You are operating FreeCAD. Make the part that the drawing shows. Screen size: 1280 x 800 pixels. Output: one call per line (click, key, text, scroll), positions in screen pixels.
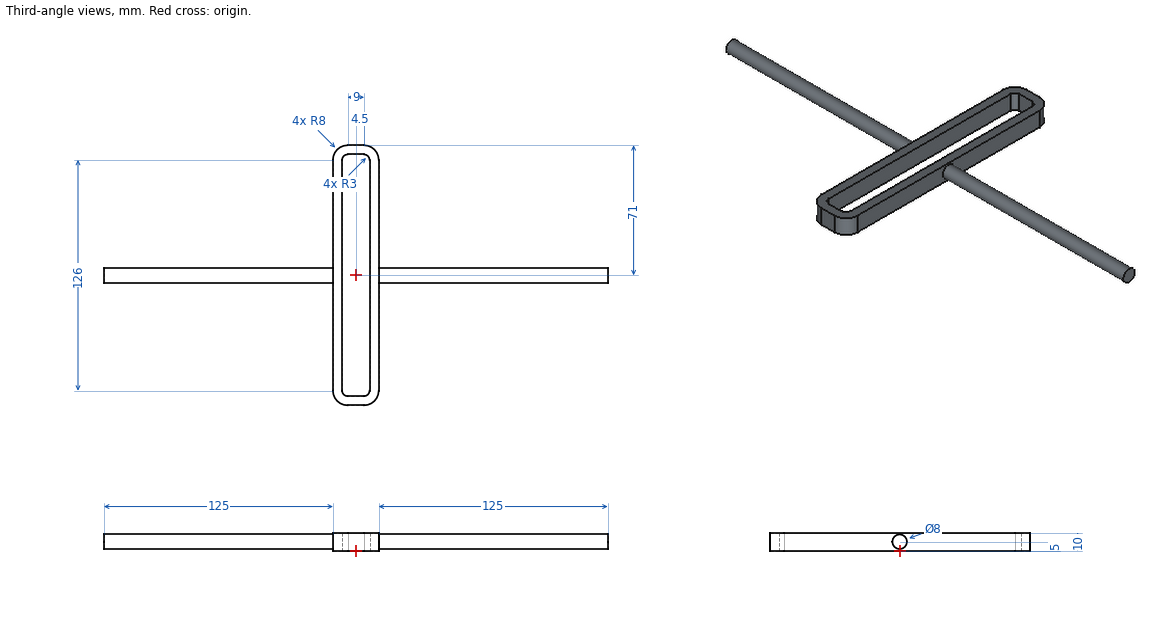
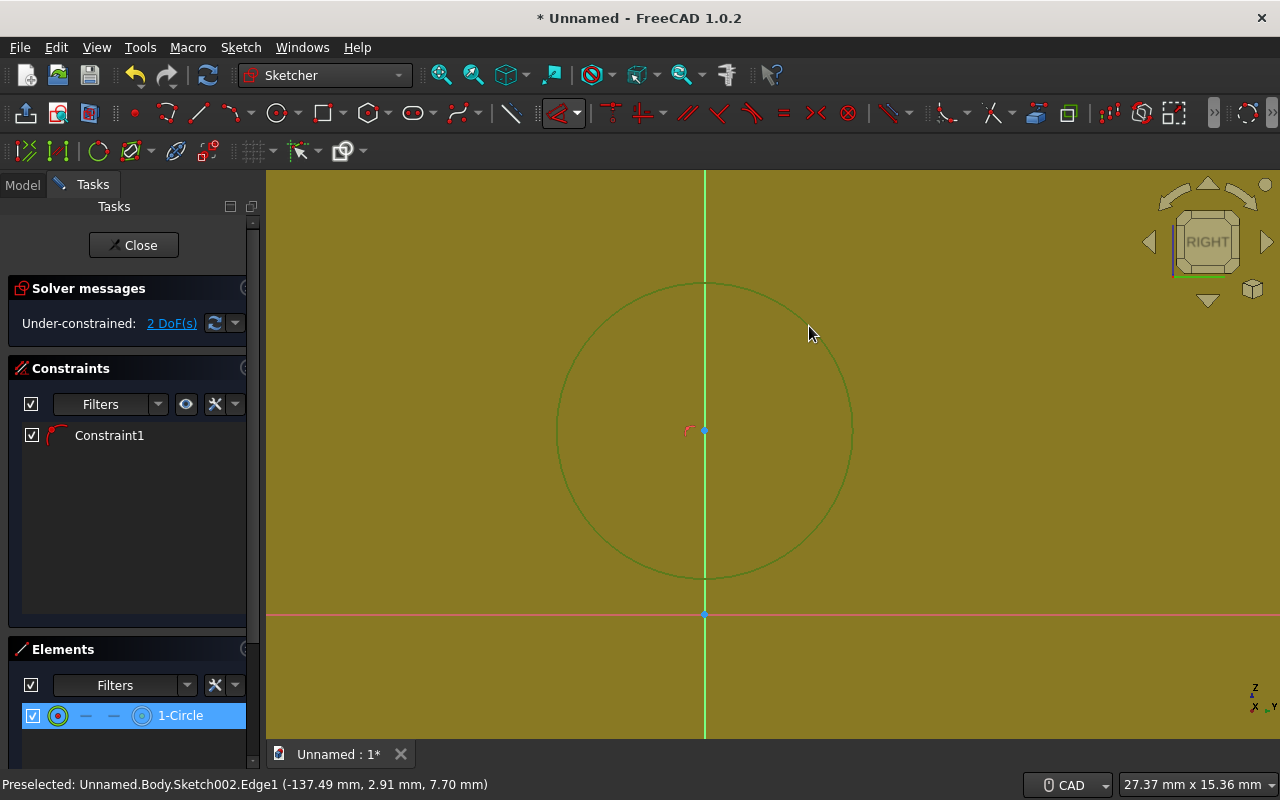
click(580, 114)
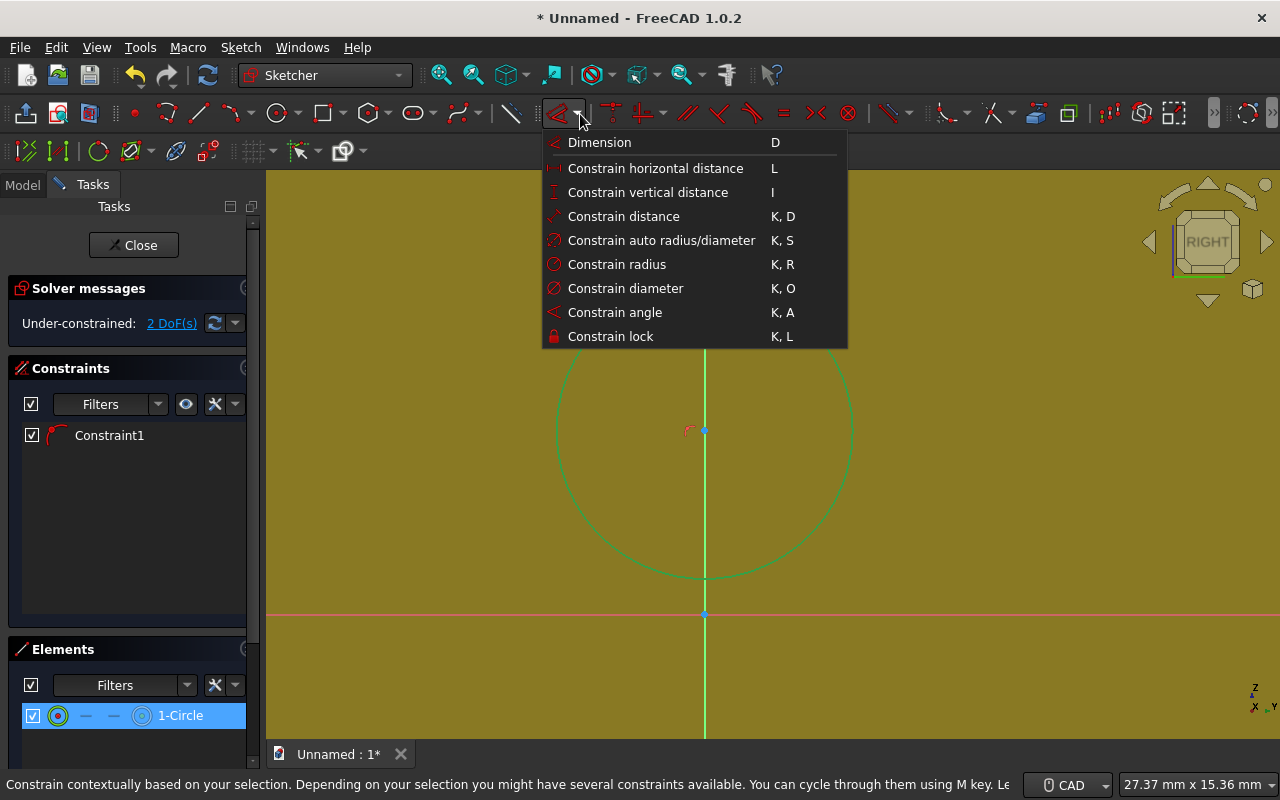
click(695, 288)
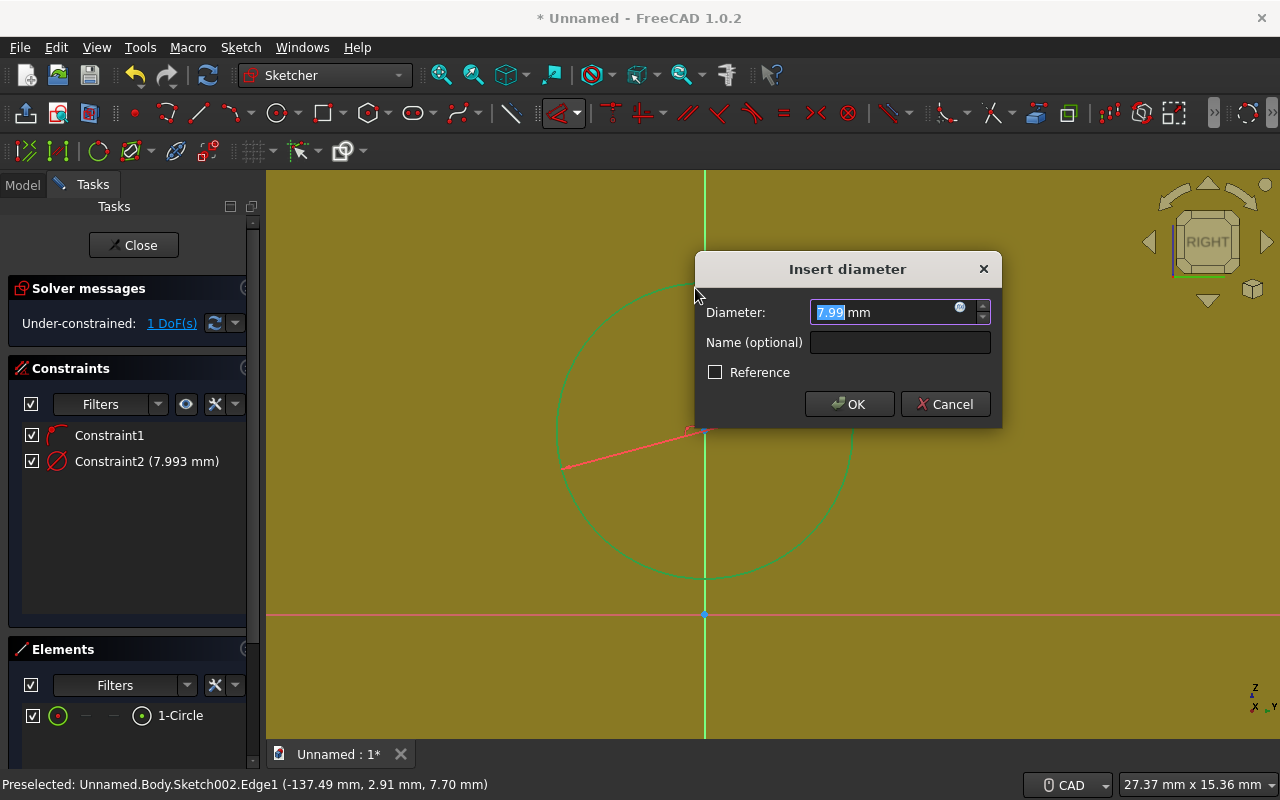
text(8)
key(Return)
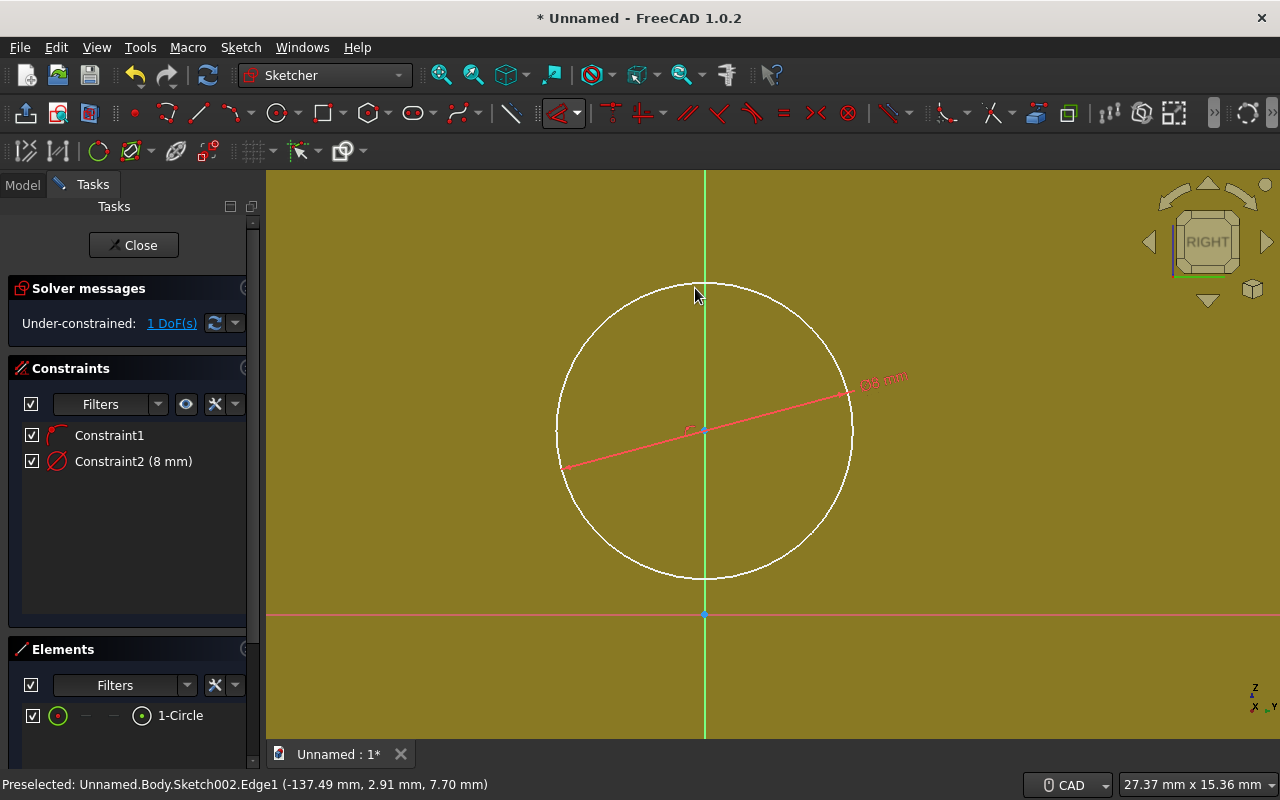
click(705, 431)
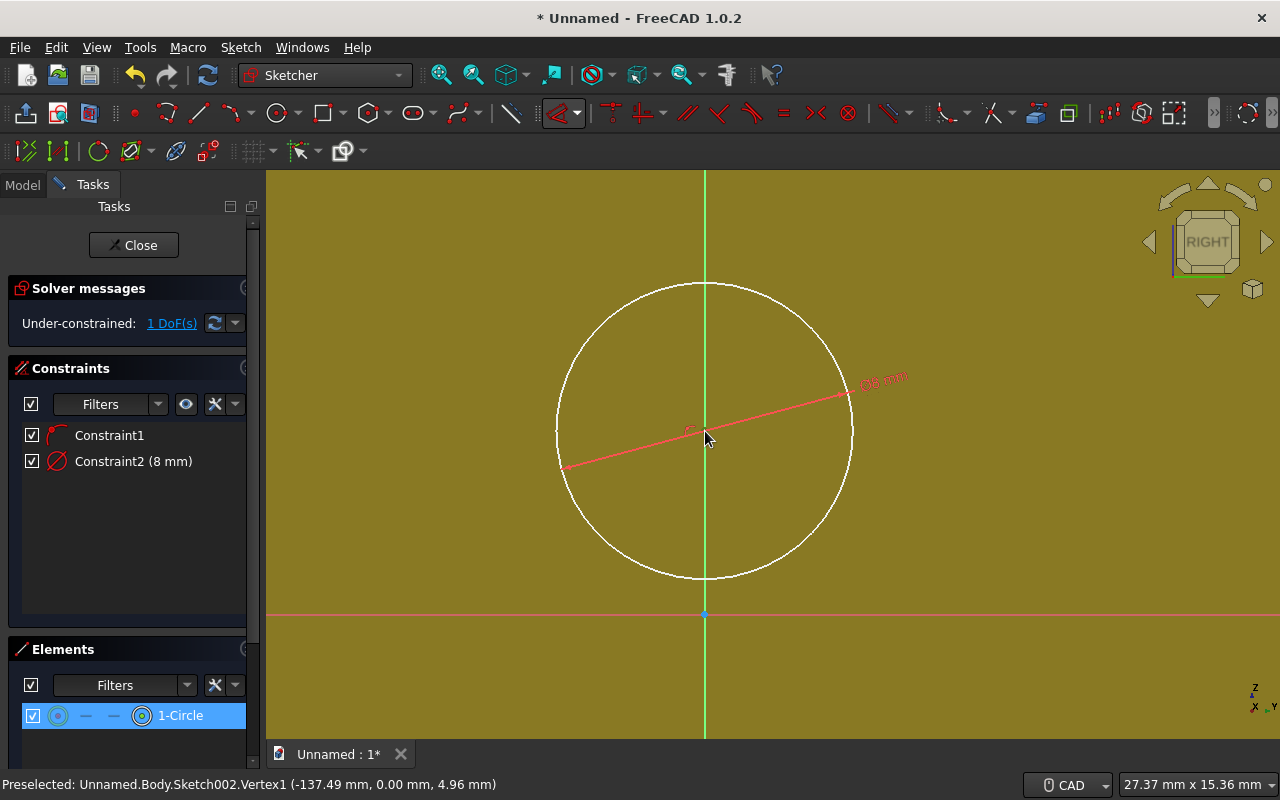
click(580, 114)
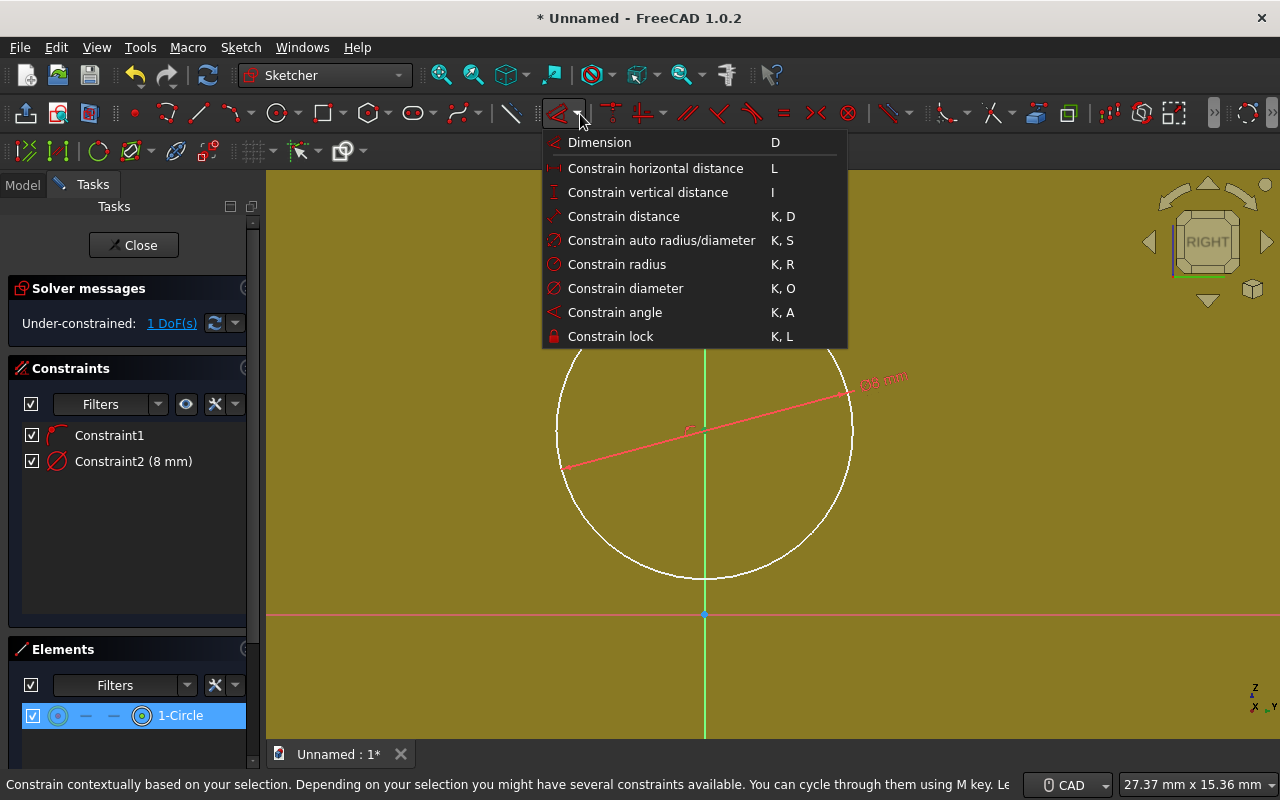
click(695, 192)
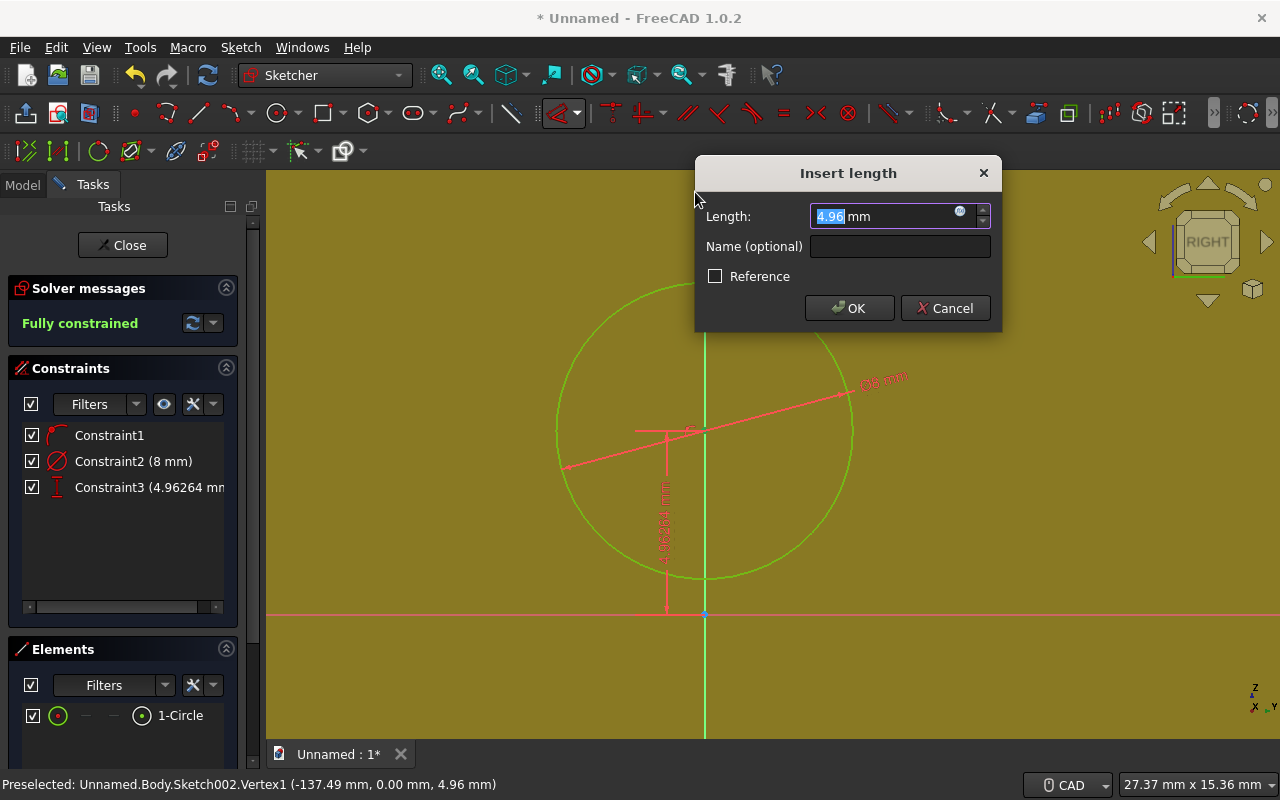
text(5)
key(Return)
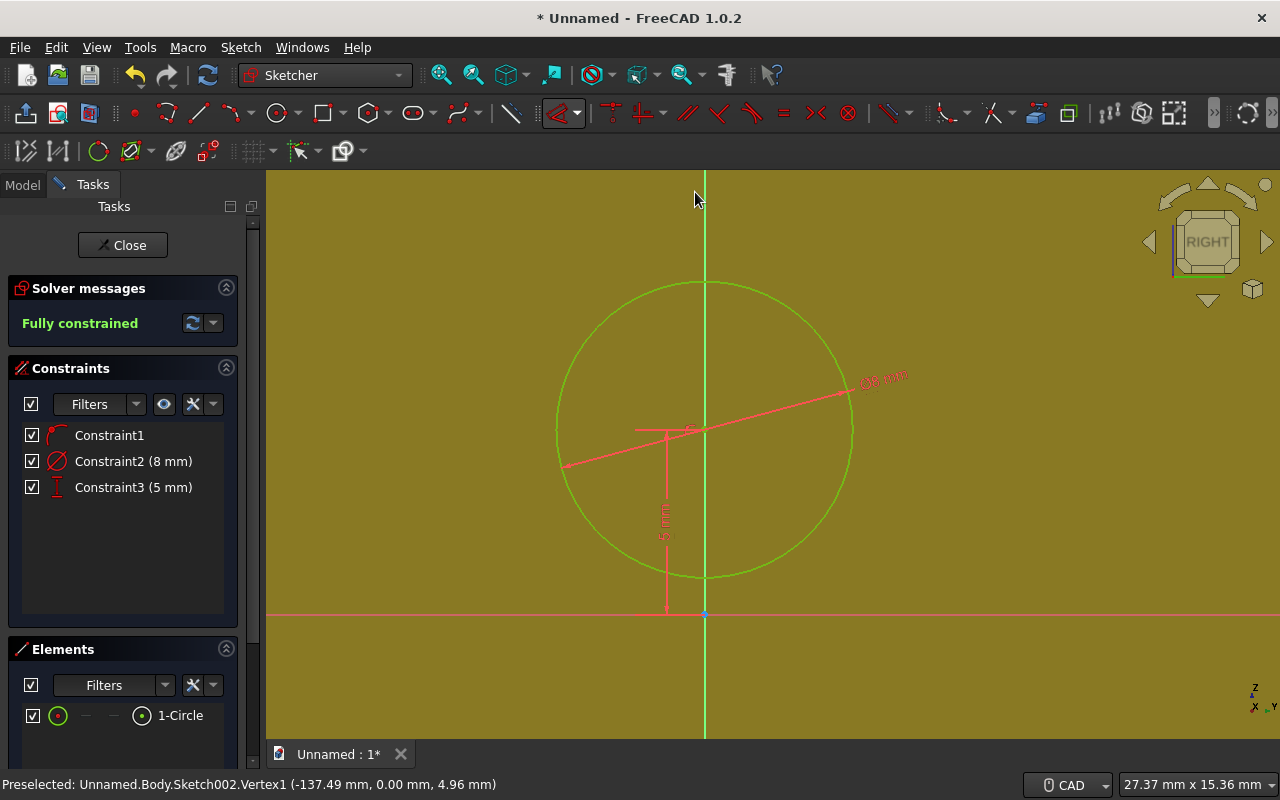
click(123, 245)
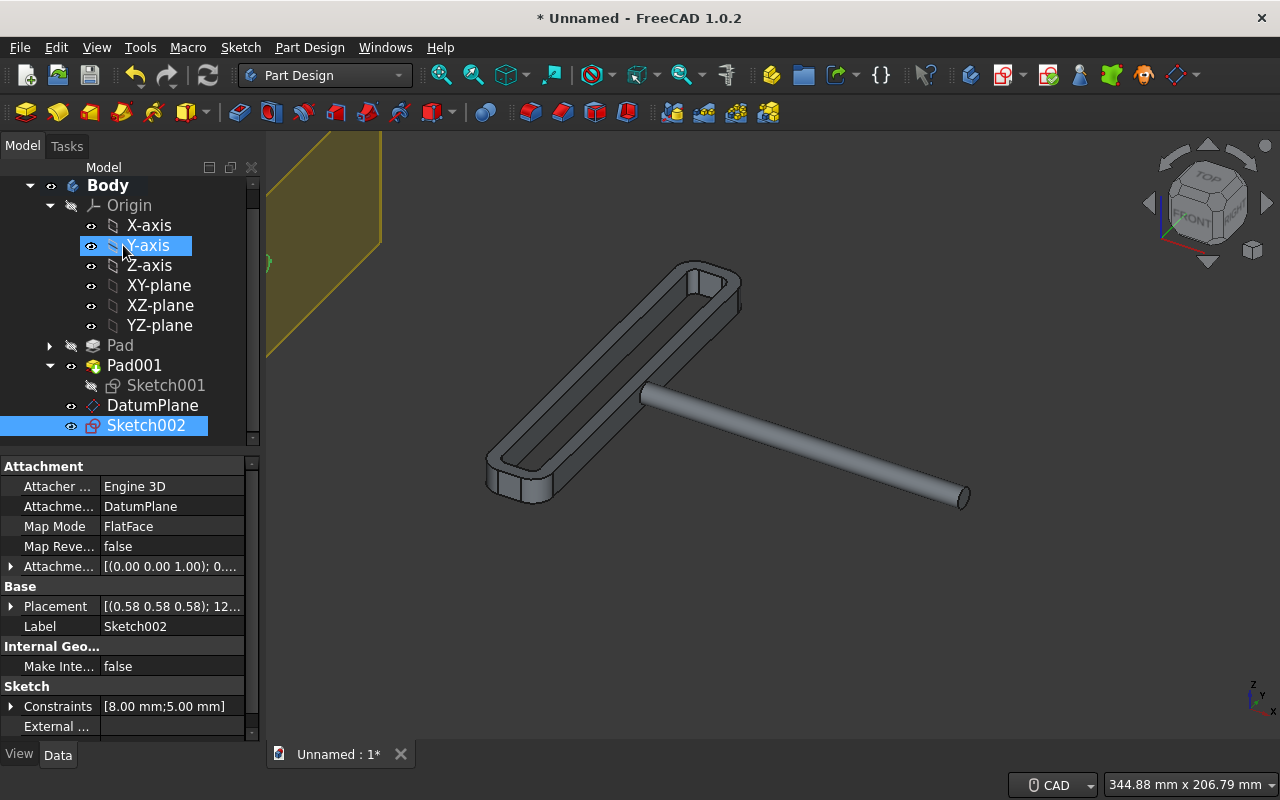
click(26, 112)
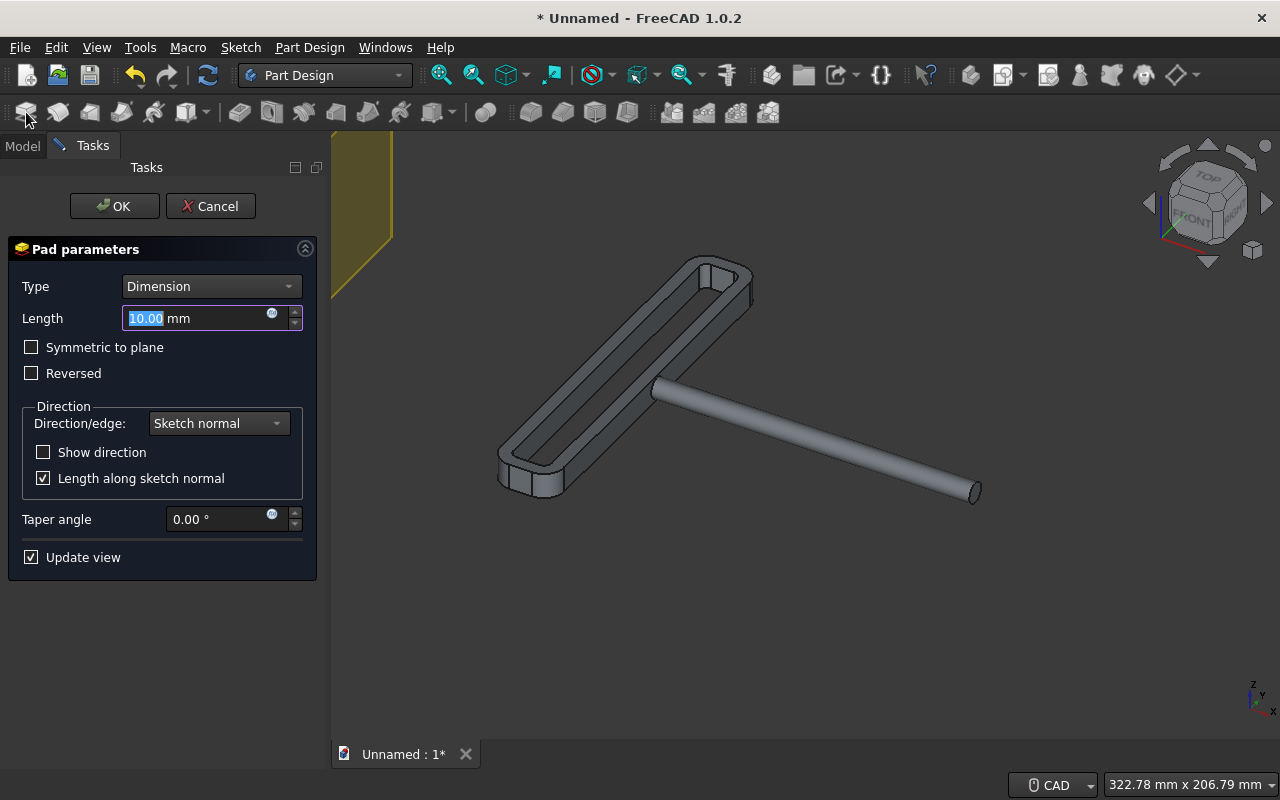
text(125)
key(Tab)